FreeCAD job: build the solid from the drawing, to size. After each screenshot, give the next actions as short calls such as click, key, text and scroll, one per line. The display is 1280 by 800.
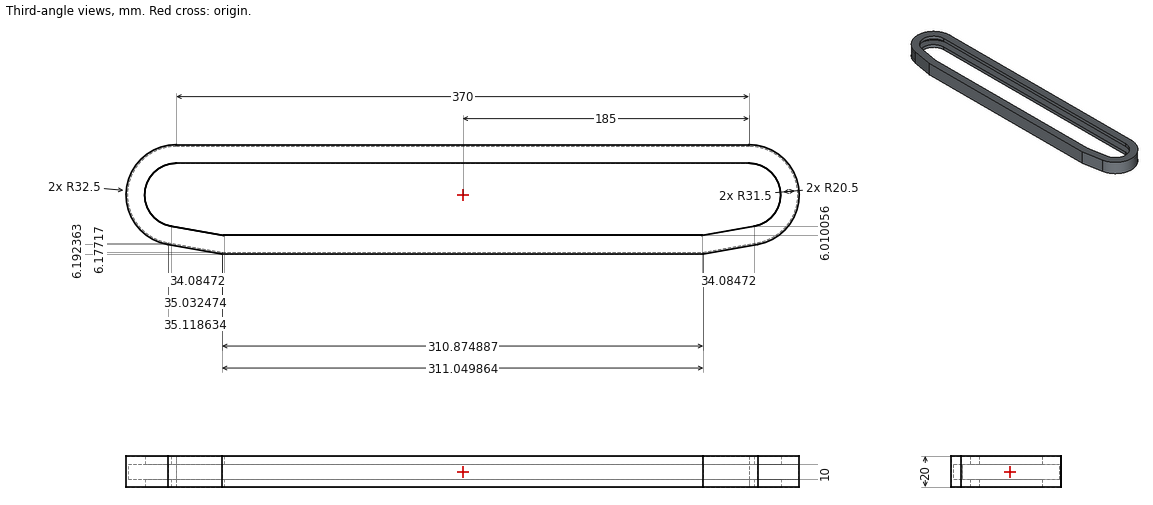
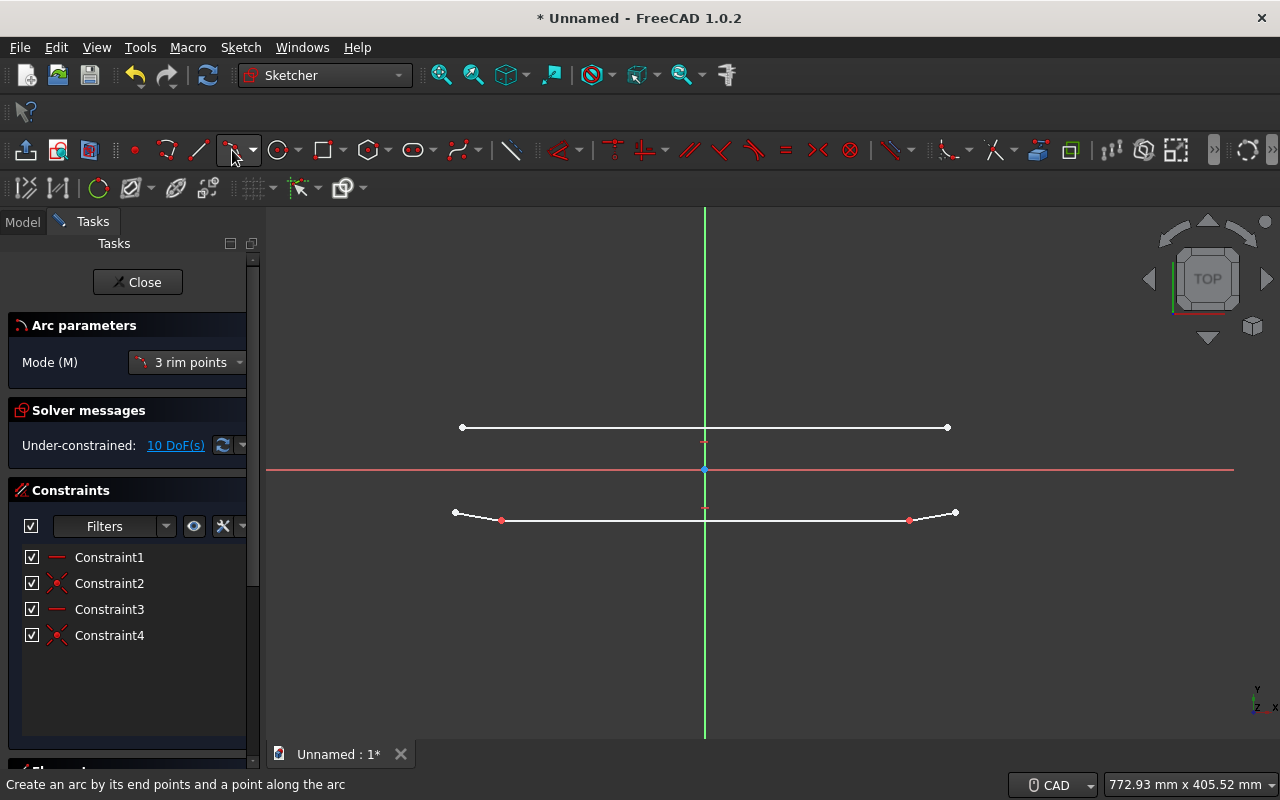
click(462, 428)
click(455, 513)
click(423, 454)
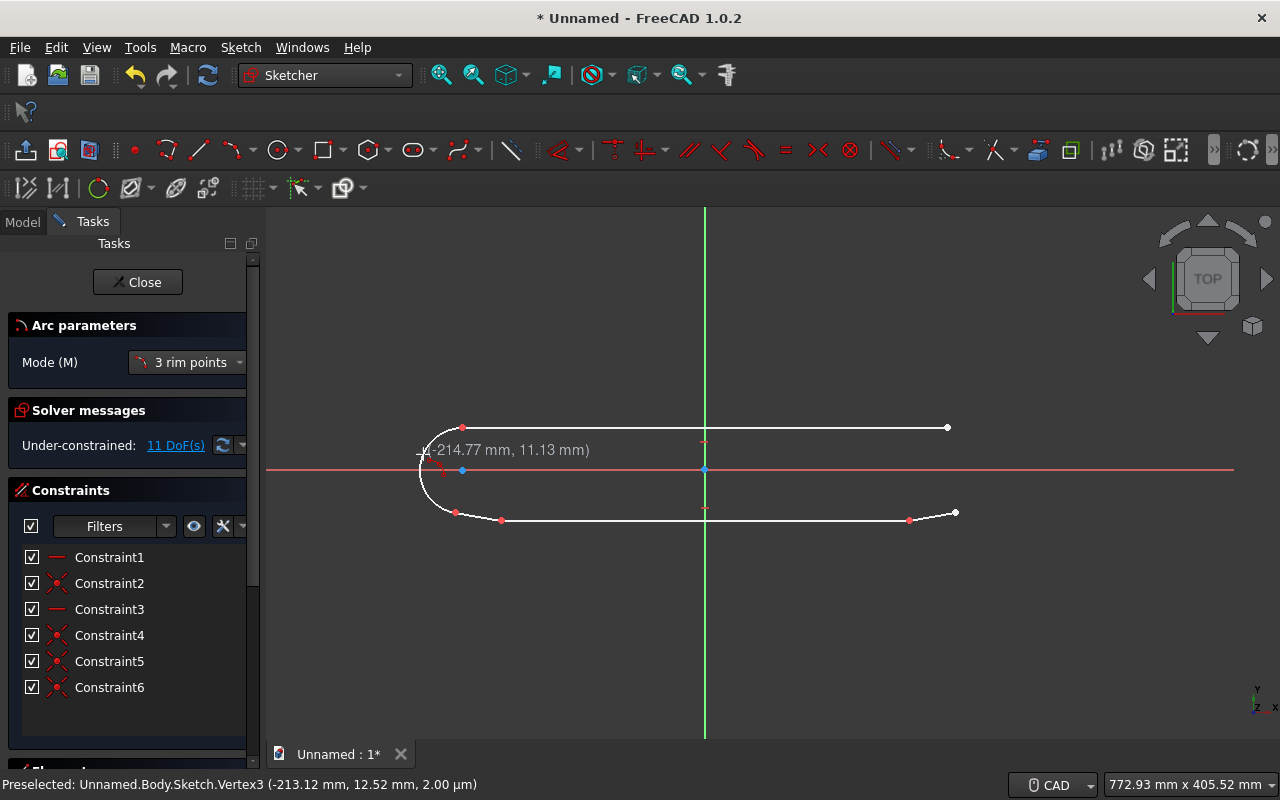
click(955, 513)
click(947, 428)
click(987, 454)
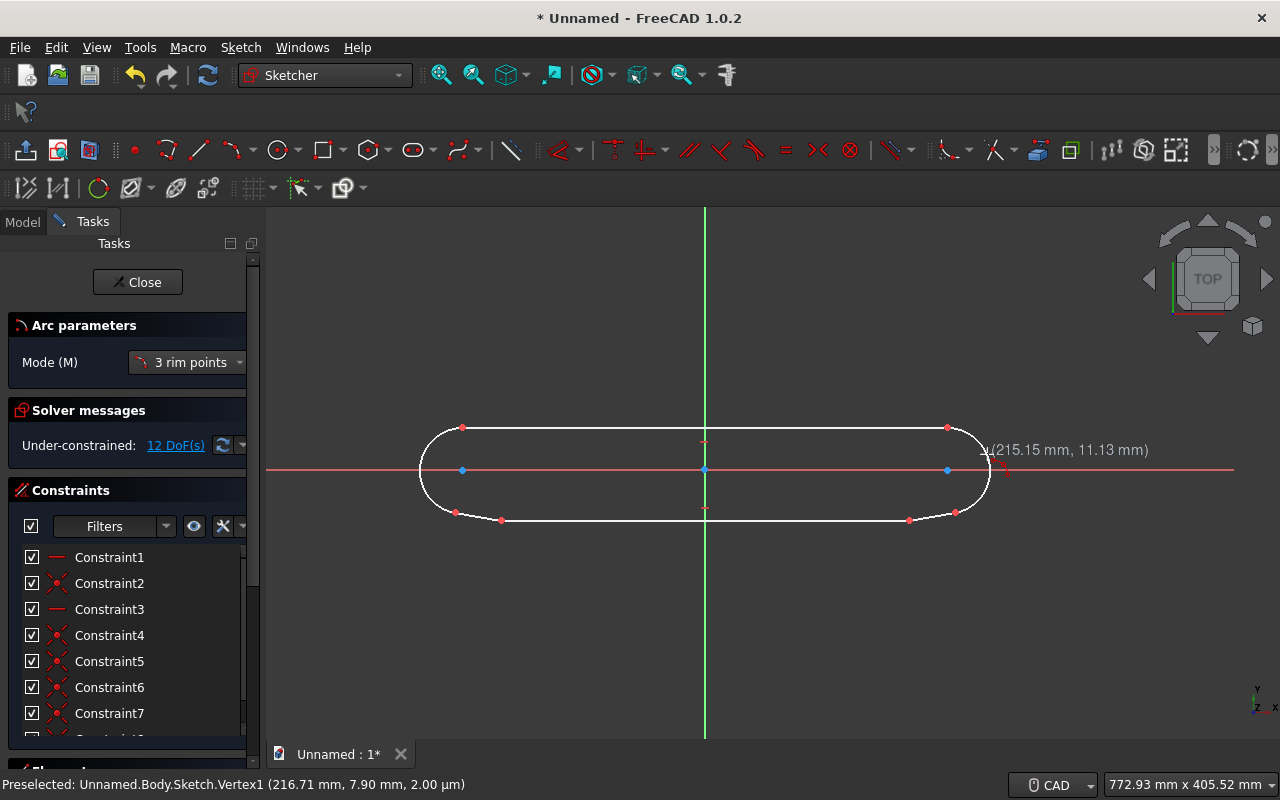
key(g)
key(l)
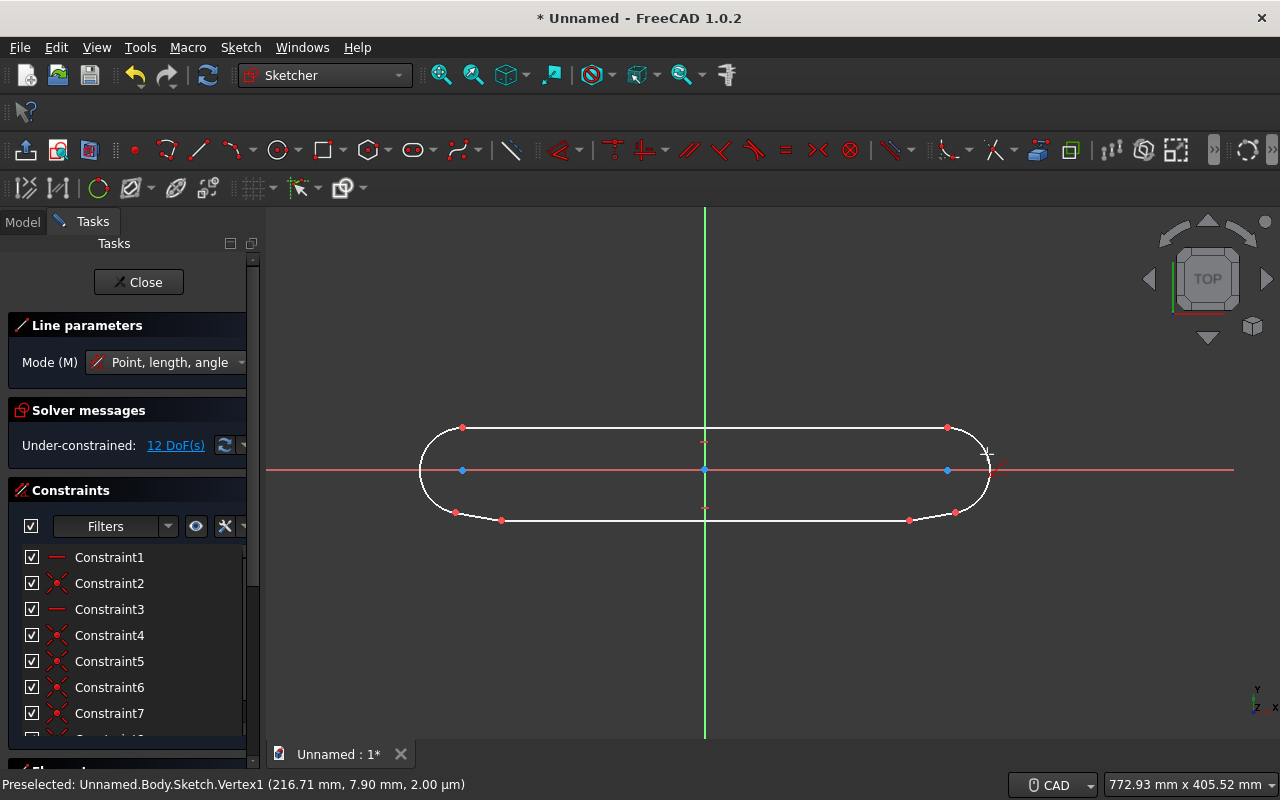
click(462, 443)
click(947, 443)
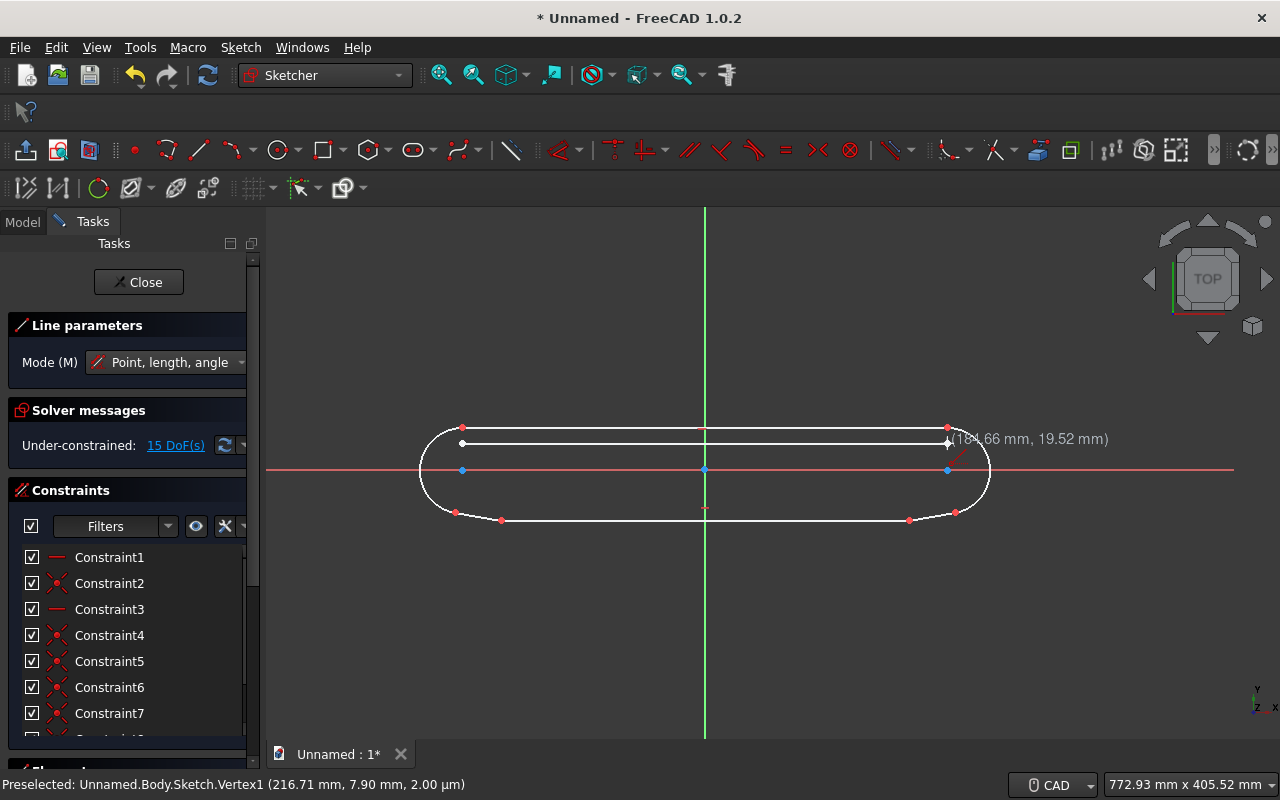
key(g)
key(m)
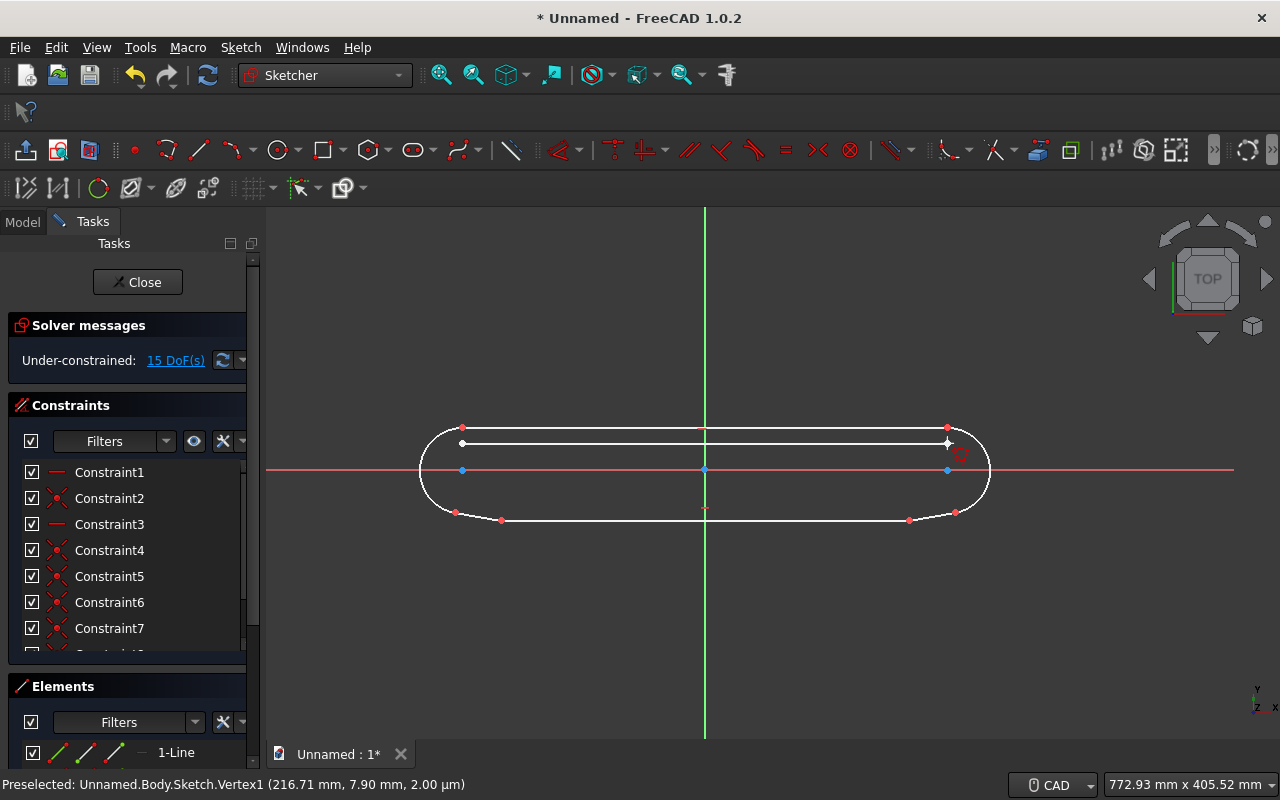
click(952, 496)
click(907, 504)
click(502, 504)
click(457, 496)
right_click(457, 496)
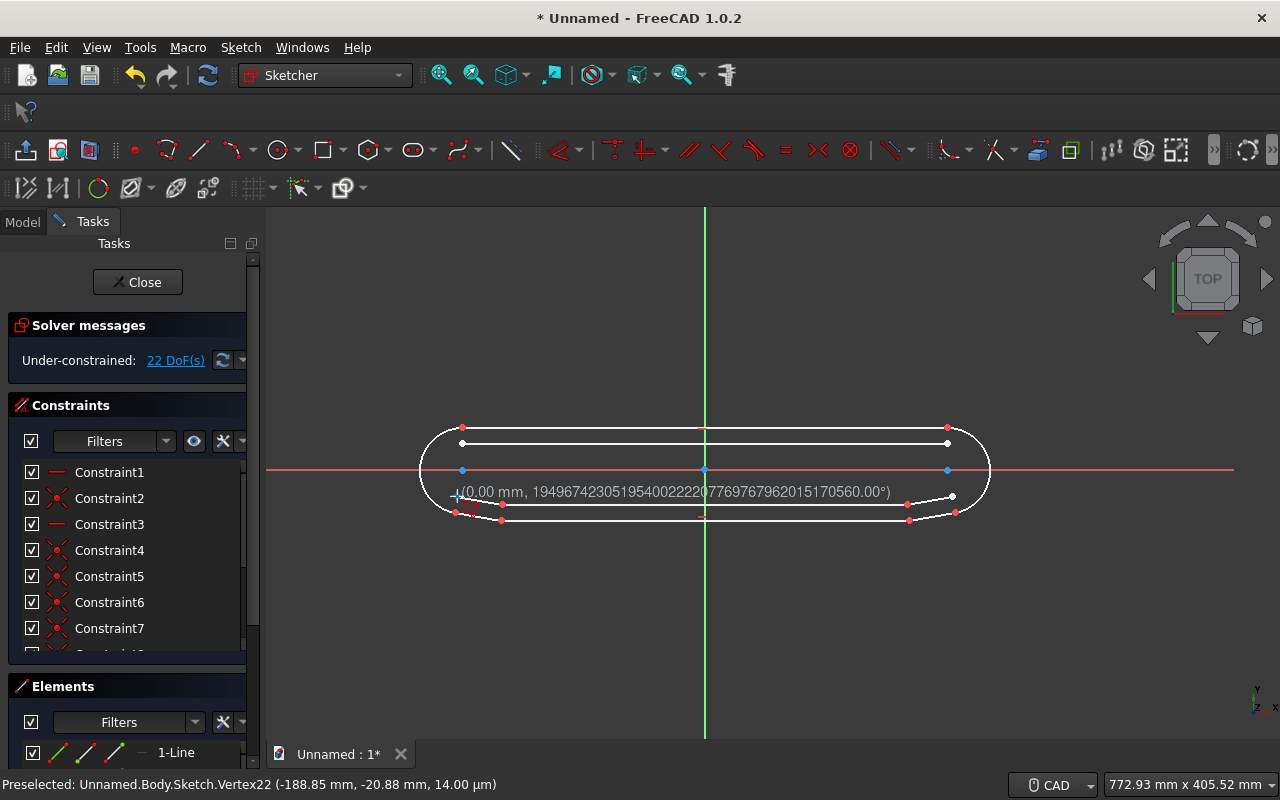
key(g)
key(3)
key(a)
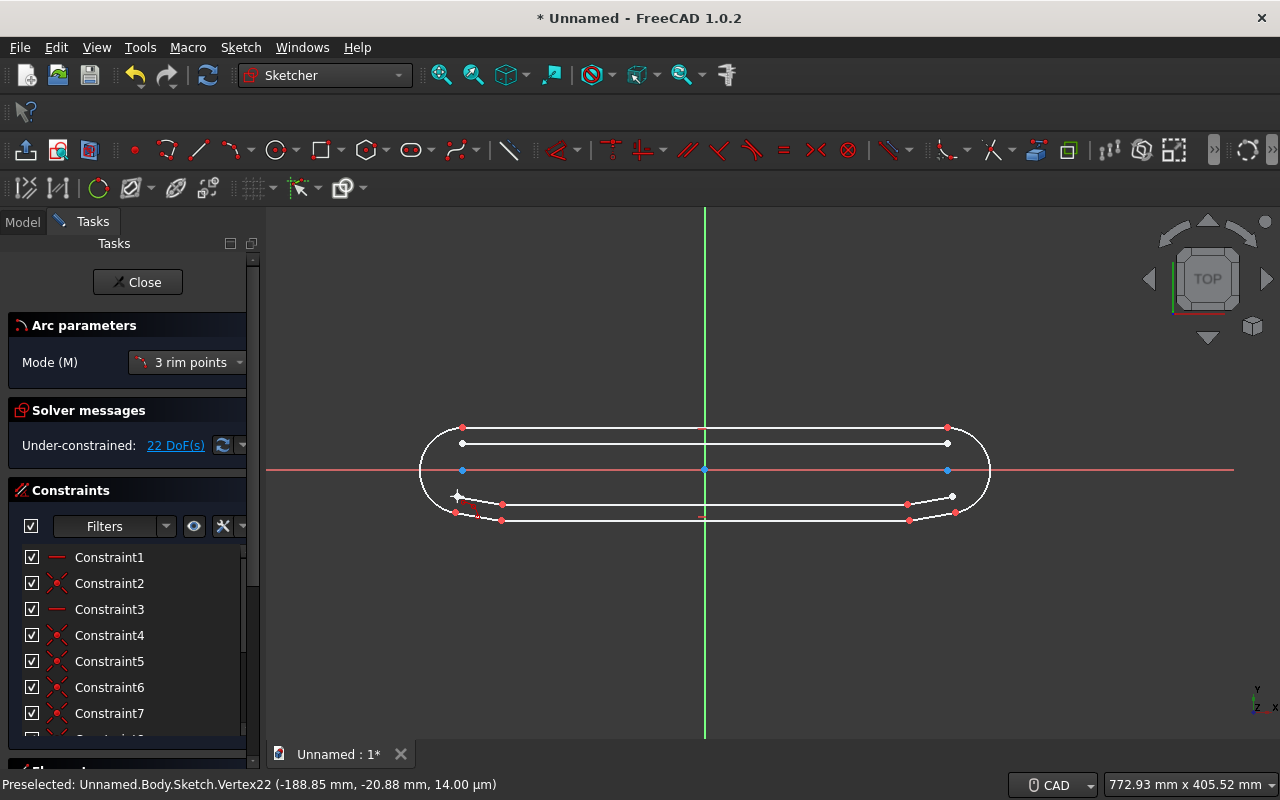
click(947, 444)
click(952, 497)
click(968, 453)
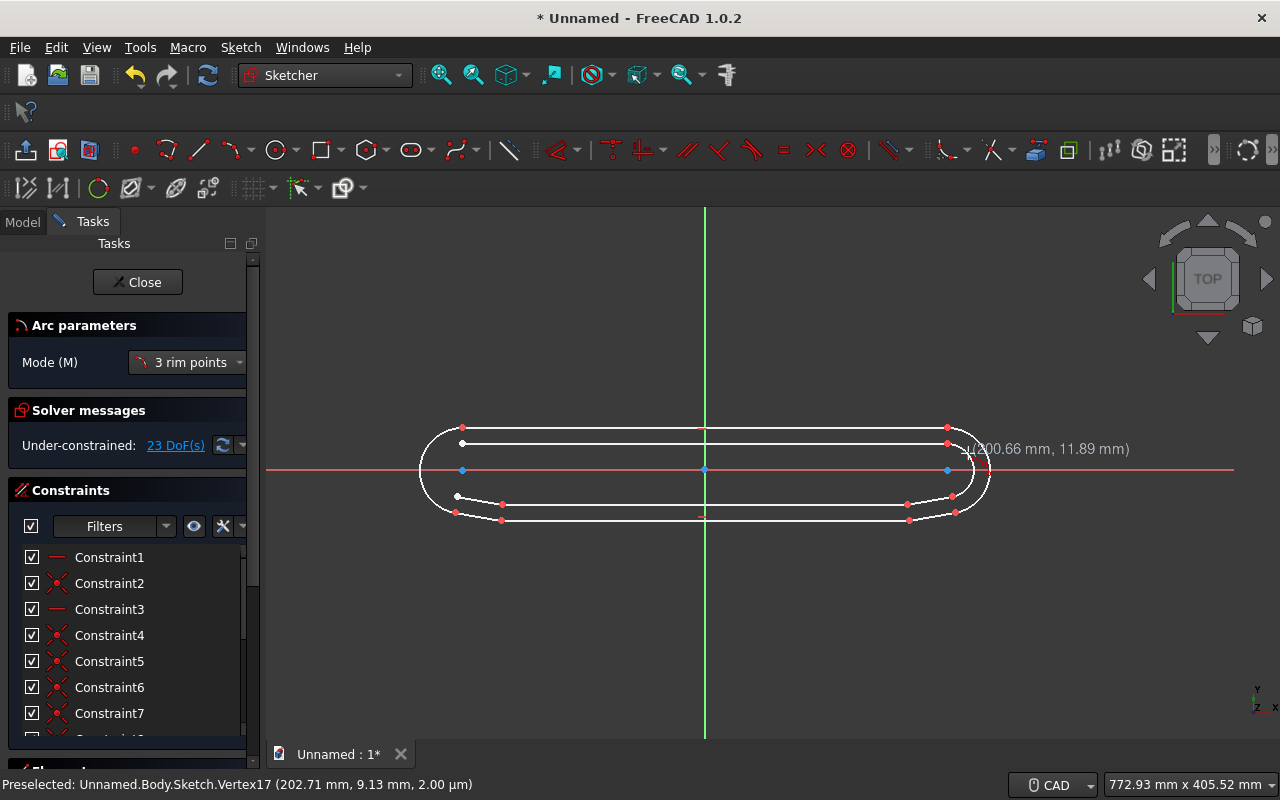
click(457, 497)
click(462, 444)
click(441, 453)
key(Escape)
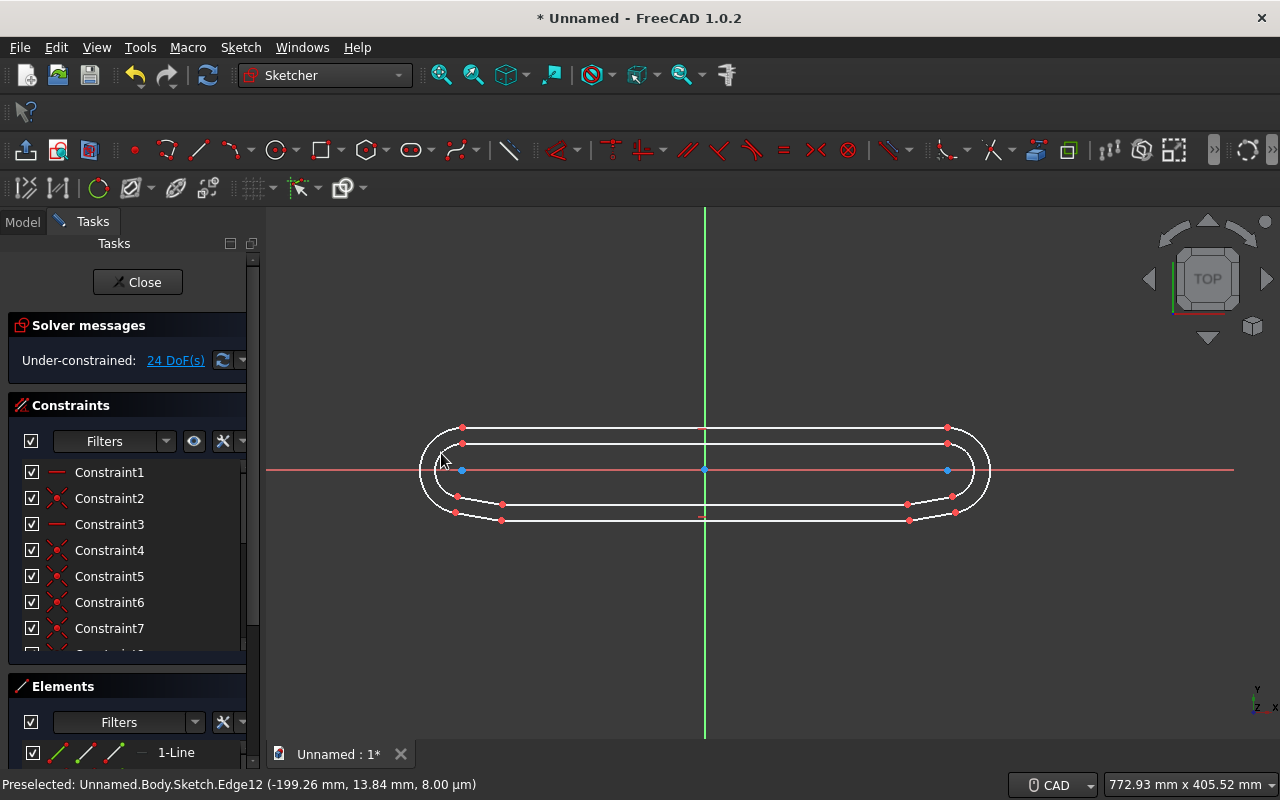
click(802, 428)